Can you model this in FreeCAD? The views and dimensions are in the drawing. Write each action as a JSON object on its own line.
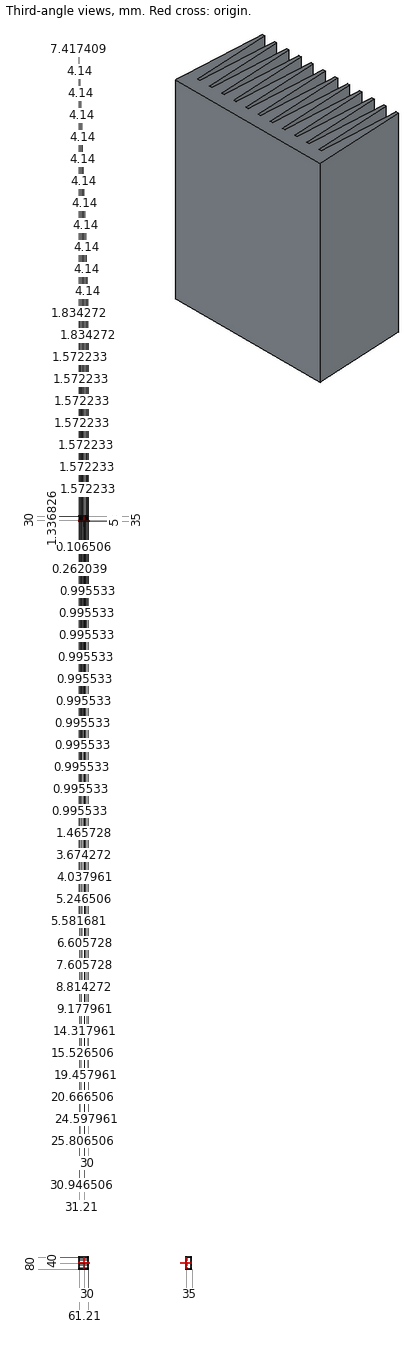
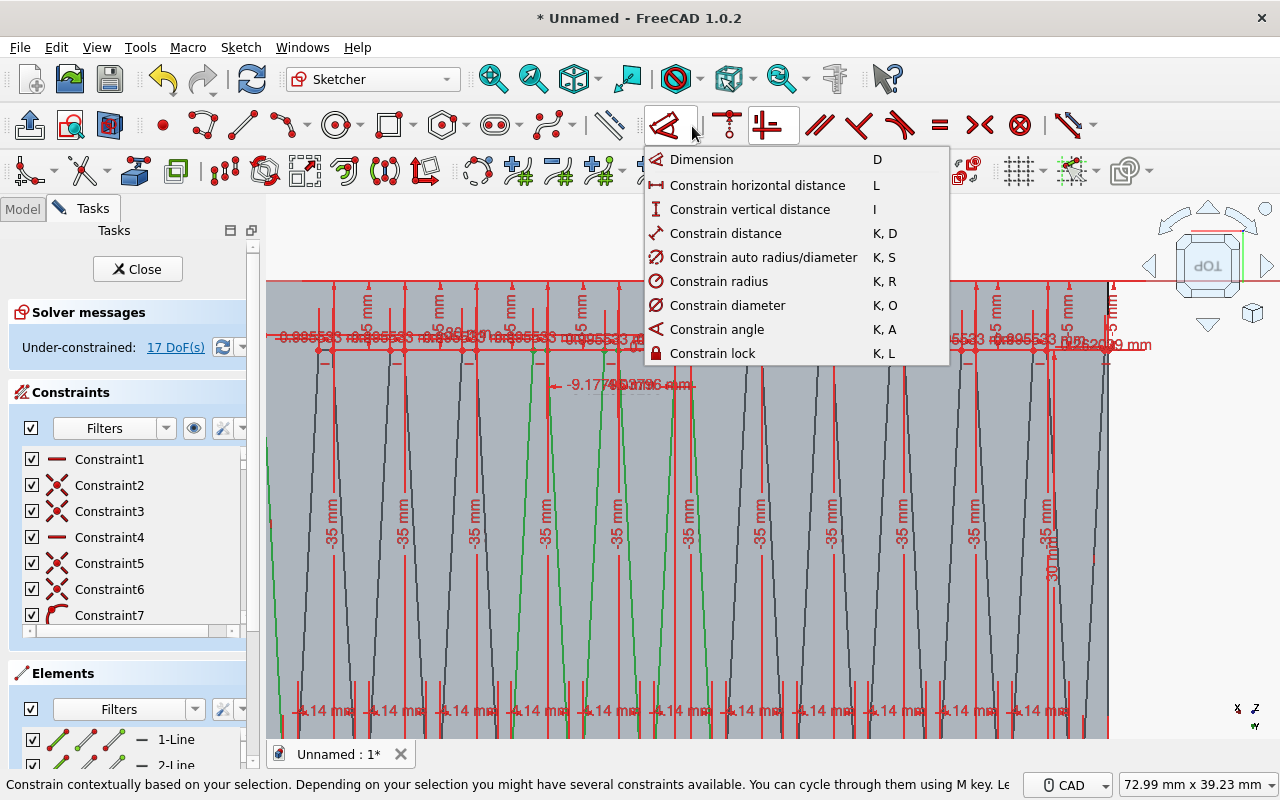
{"action": "left_click", "coordinate": [797, 185]}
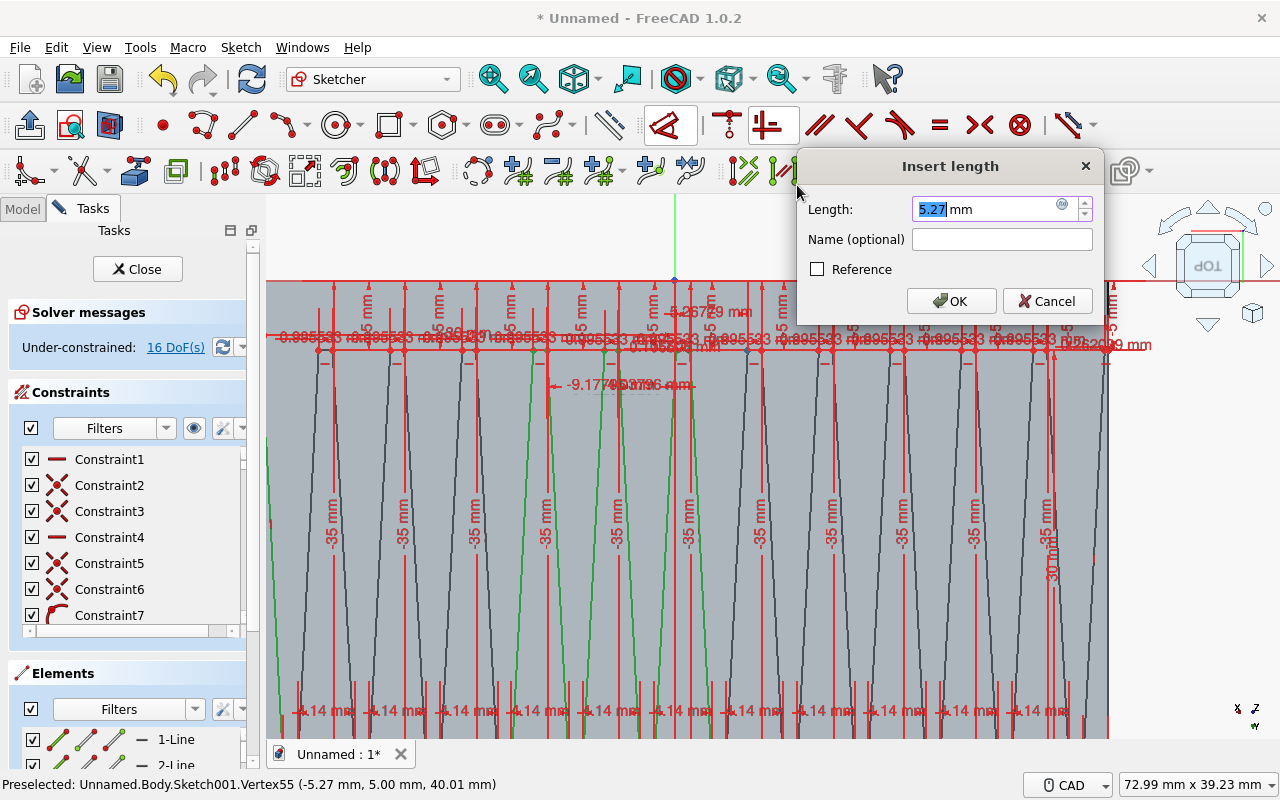
{"action": "type", "text": "5.246506"}
{"action": "key", "text": "Return"}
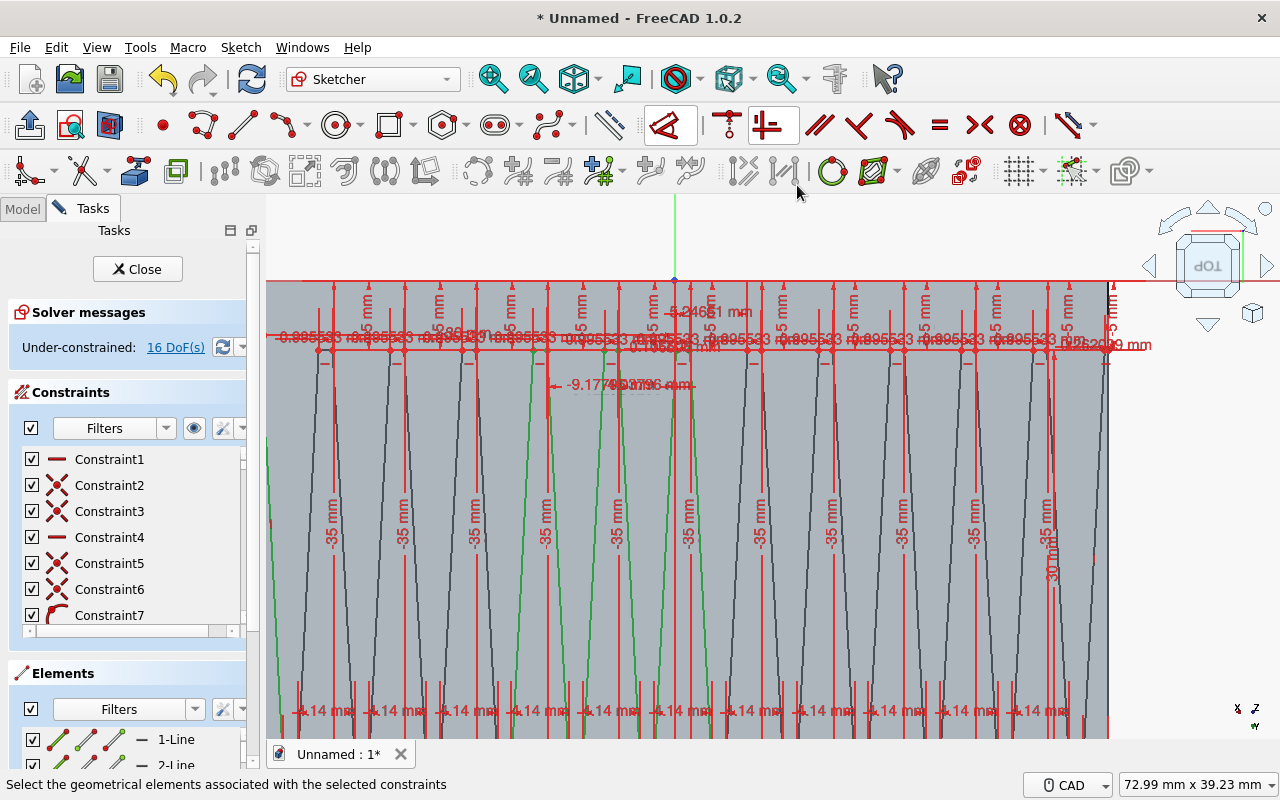
{"action": "scroll", "coordinate": [748, 350], "scroll_direction": "down", "scroll_amount": 2}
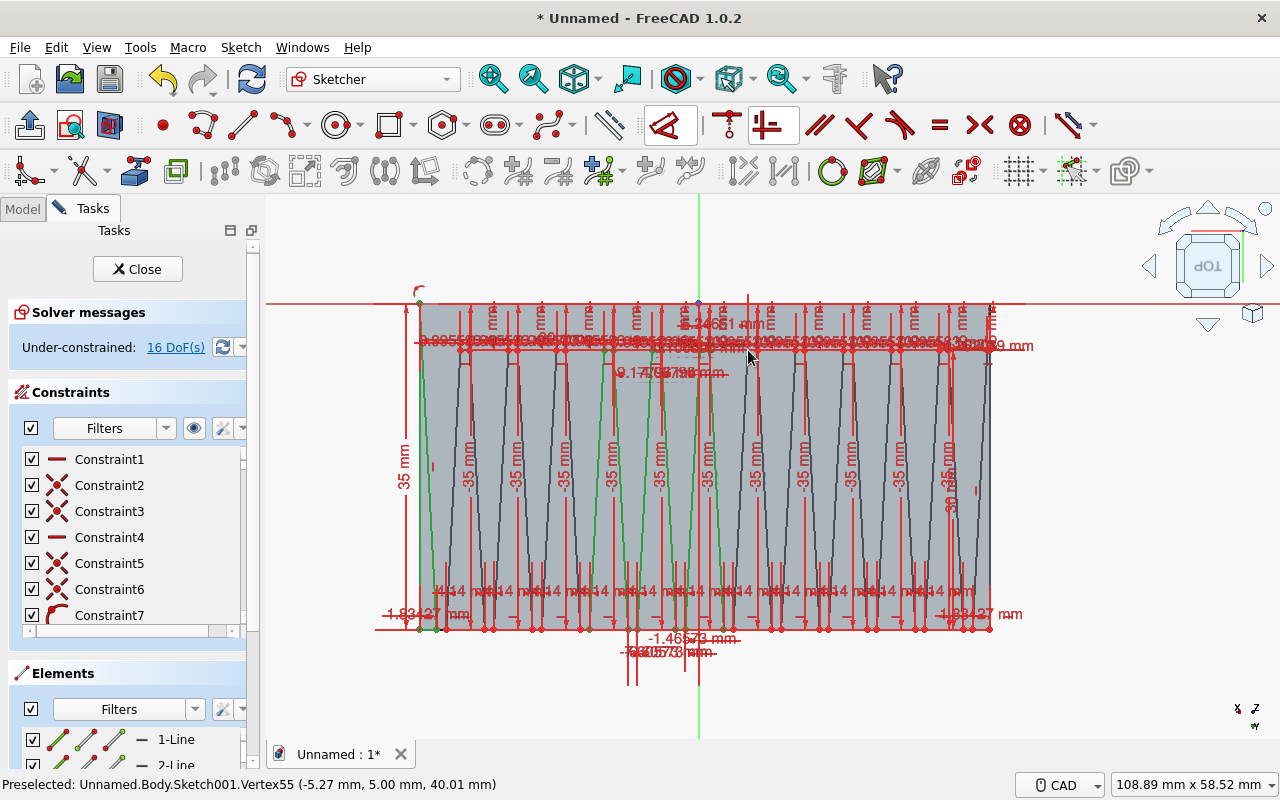
{"action": "scroll", "coordinate": [733, 630], "scroll_direction": "up", "scroll_amount": 2}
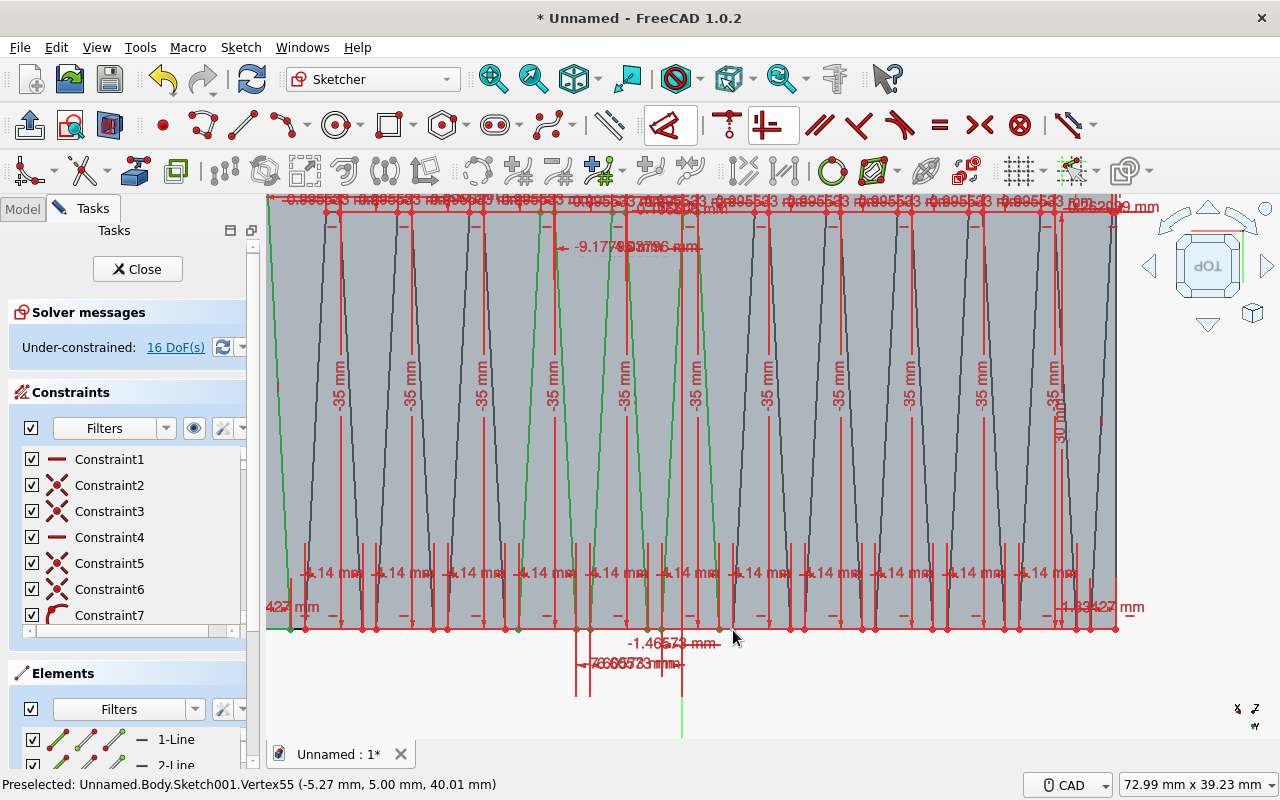
{"action": "left_click", "coordinate": [733, 629]}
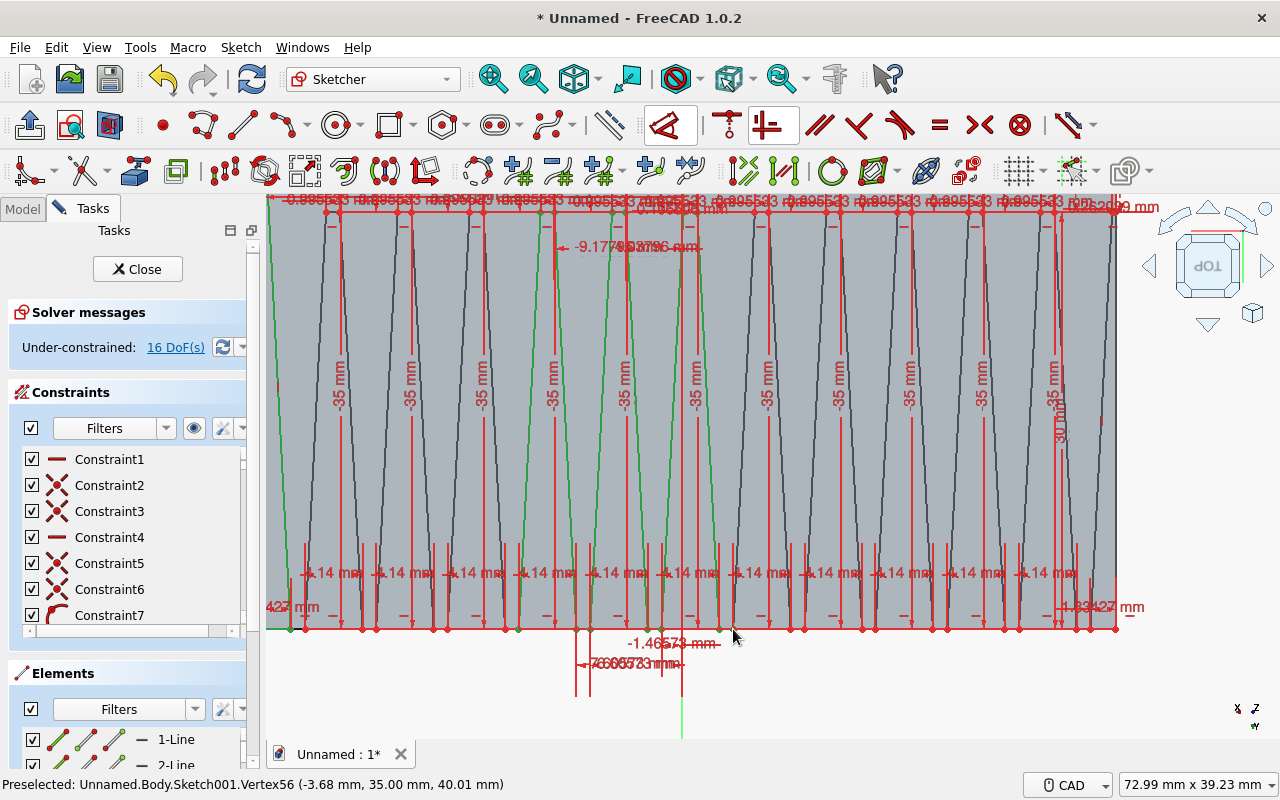
{"action": "left_click", "coordinate": [692, 126]}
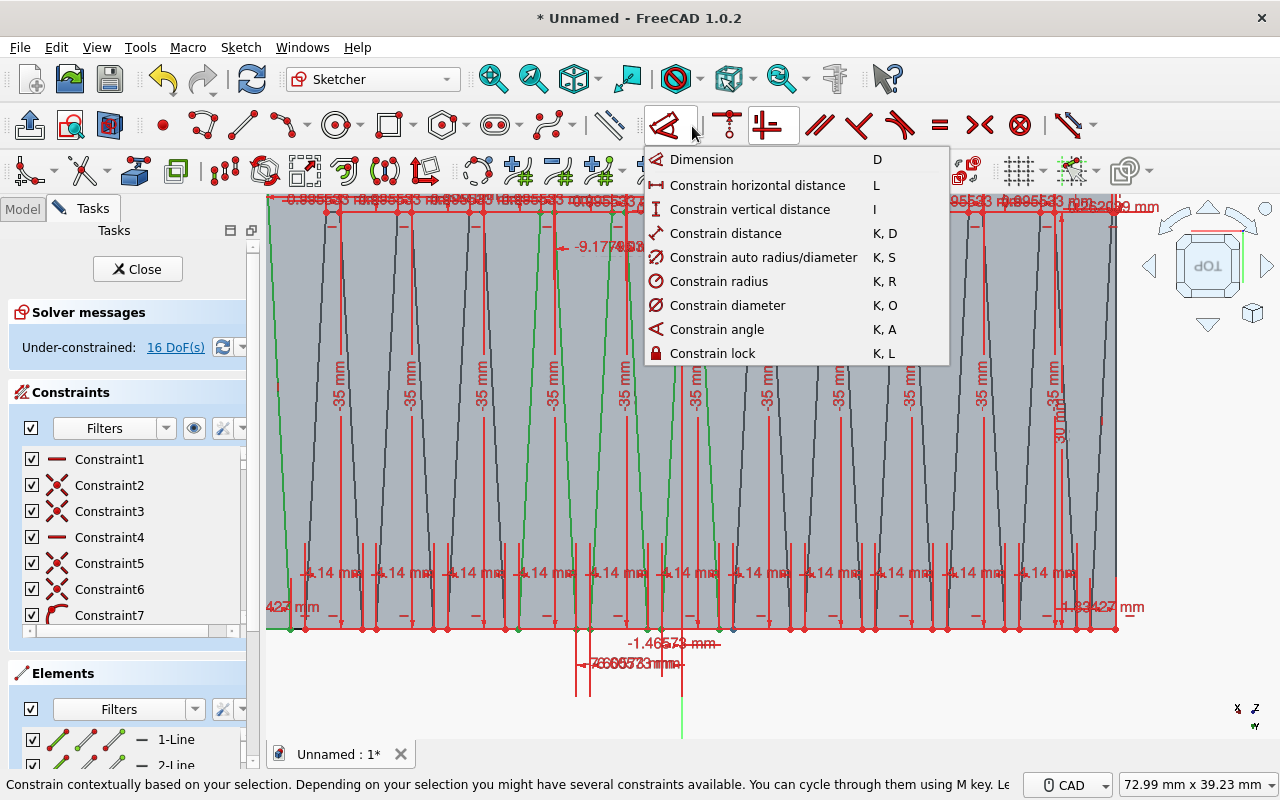
{"action": "left_click", "coordinate": [797, 185]}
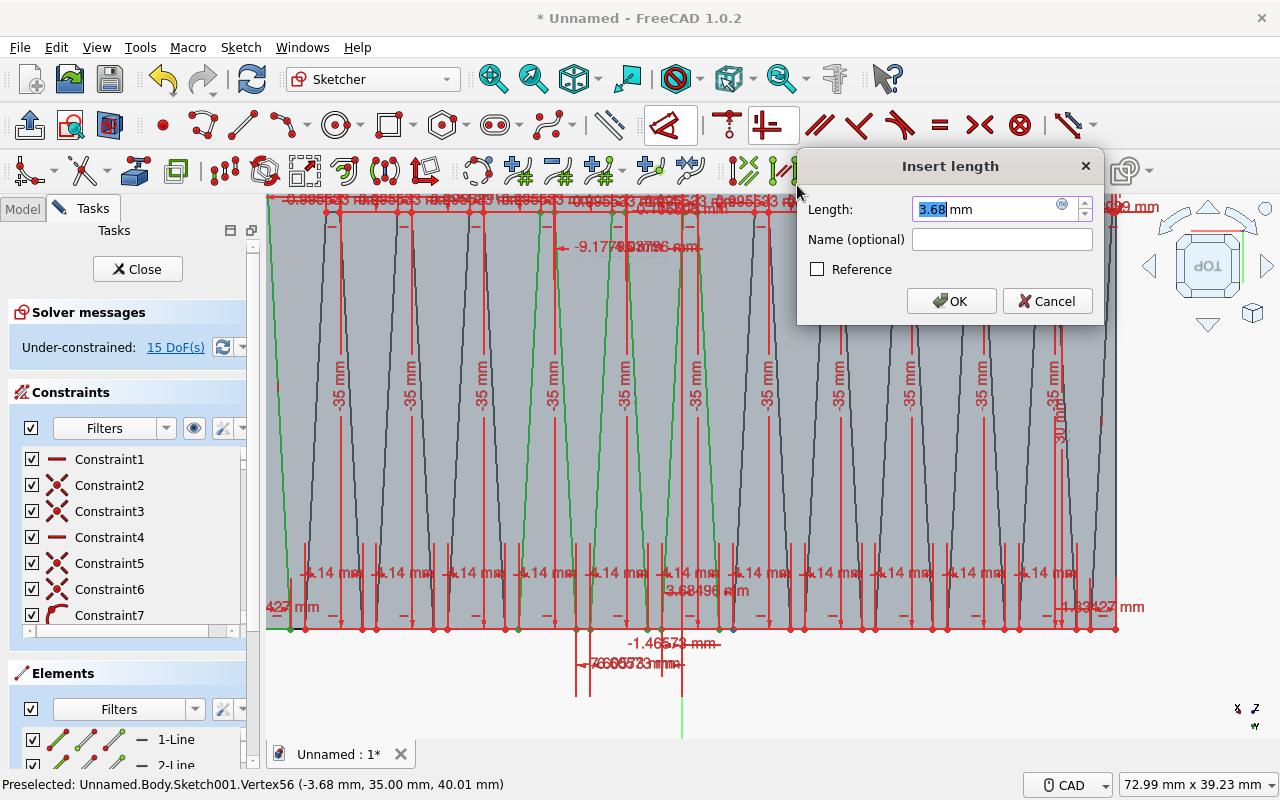
{"action": "type", "text": "3.674272"}
{"action": "key", "text": "Return"}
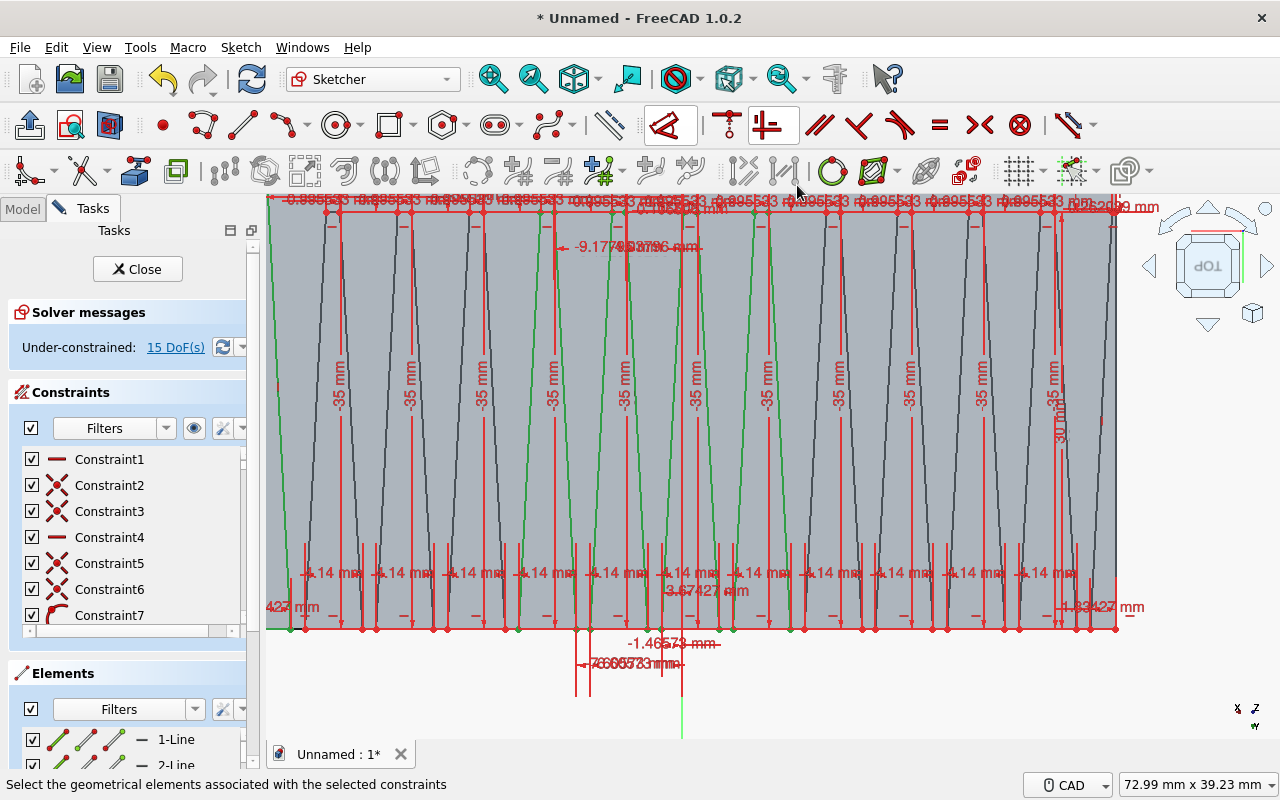
{"action": "left_click", "coordinate": [805, 629]}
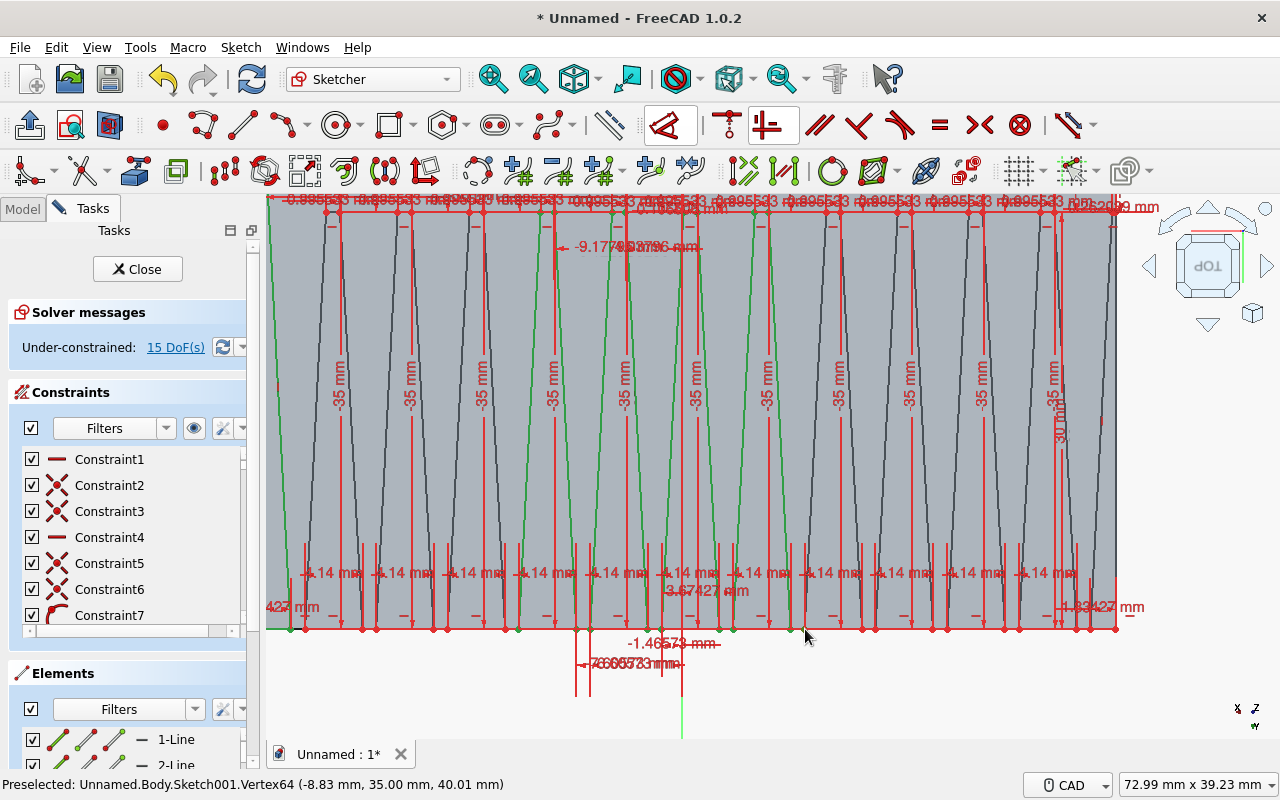
{"action": "left_click", "coordinate": [692, 126]}